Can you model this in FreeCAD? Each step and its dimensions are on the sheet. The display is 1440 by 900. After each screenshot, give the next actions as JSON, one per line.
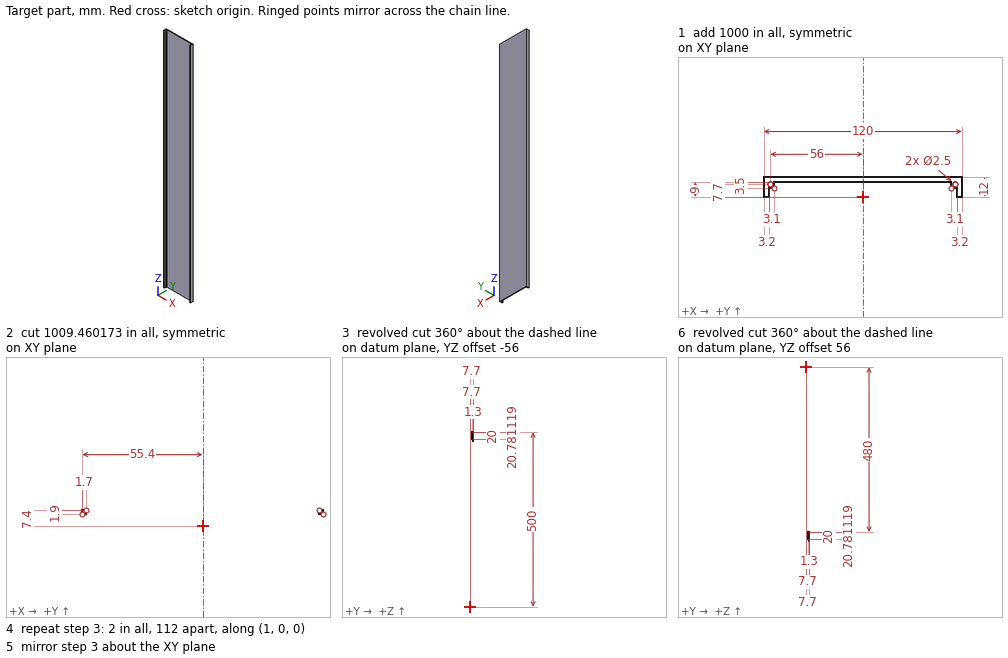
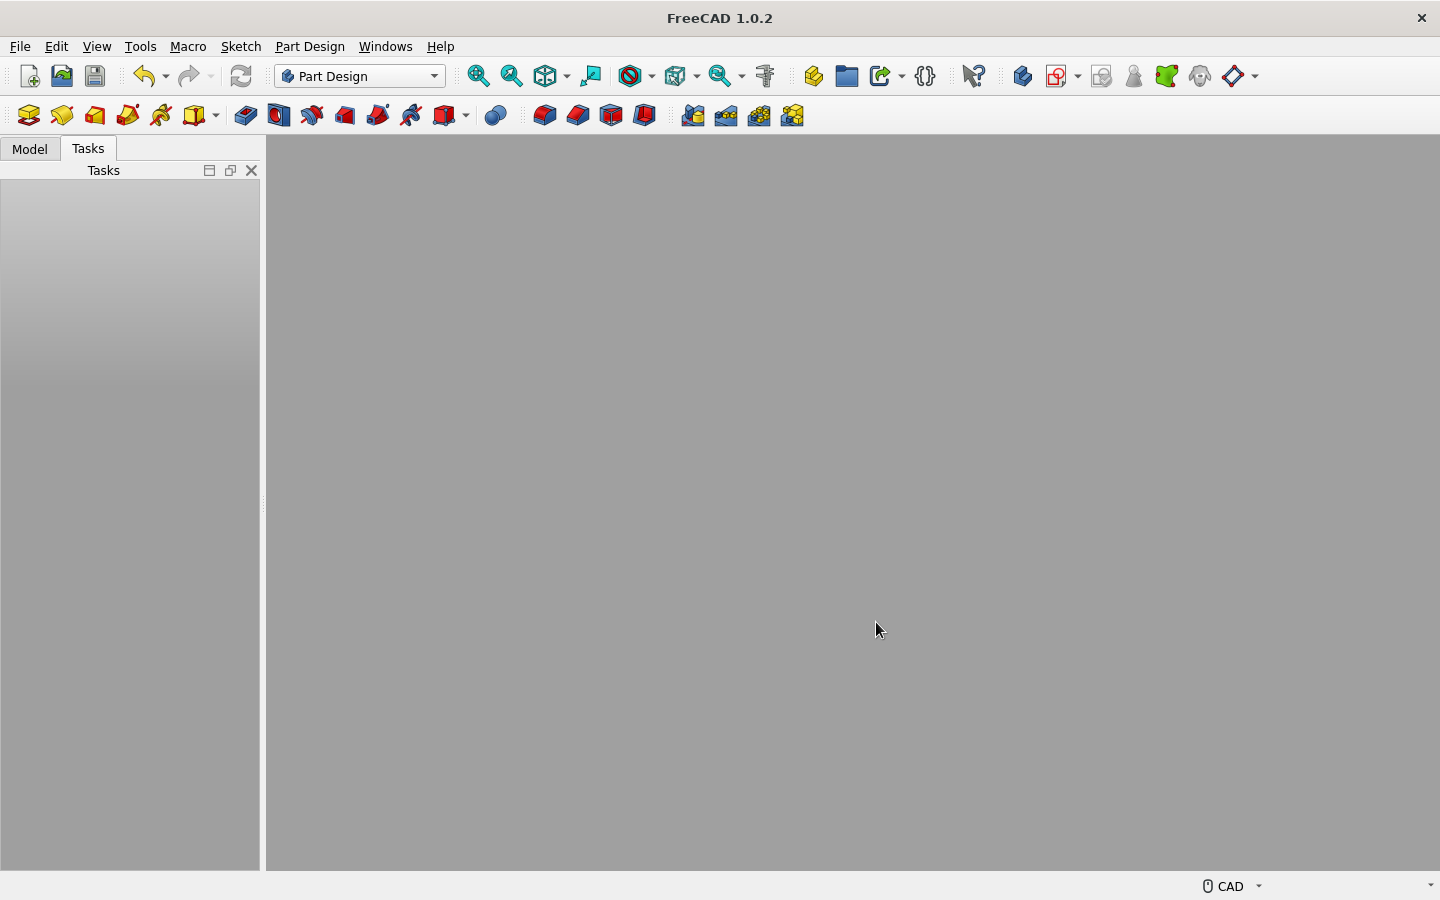
{"action": "left_click", "coordinate": [29, 76]}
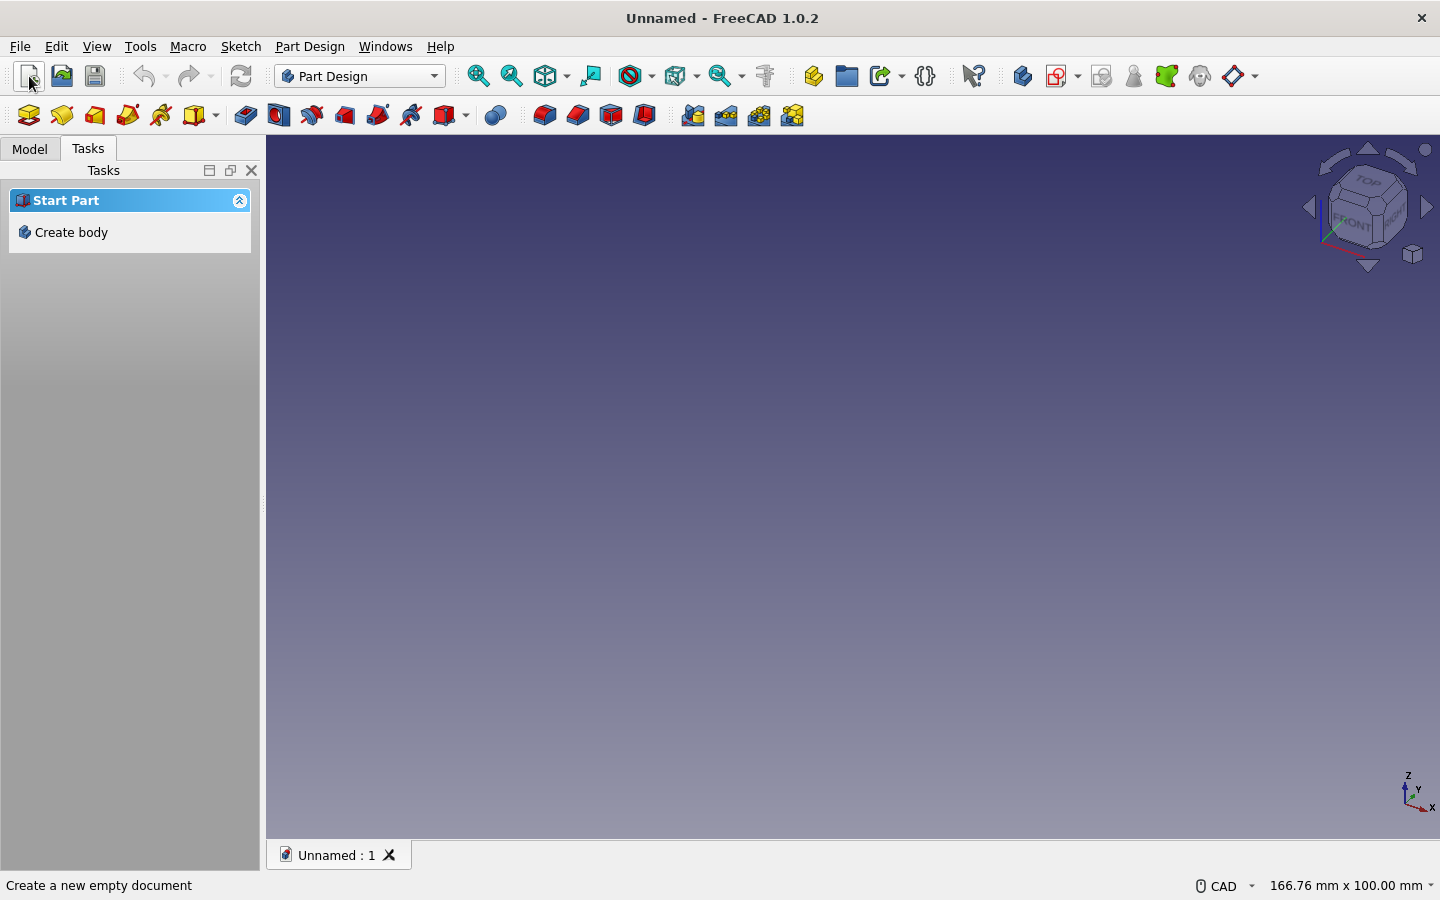
{"action": "left_click", "coordinate": [1056, 76]}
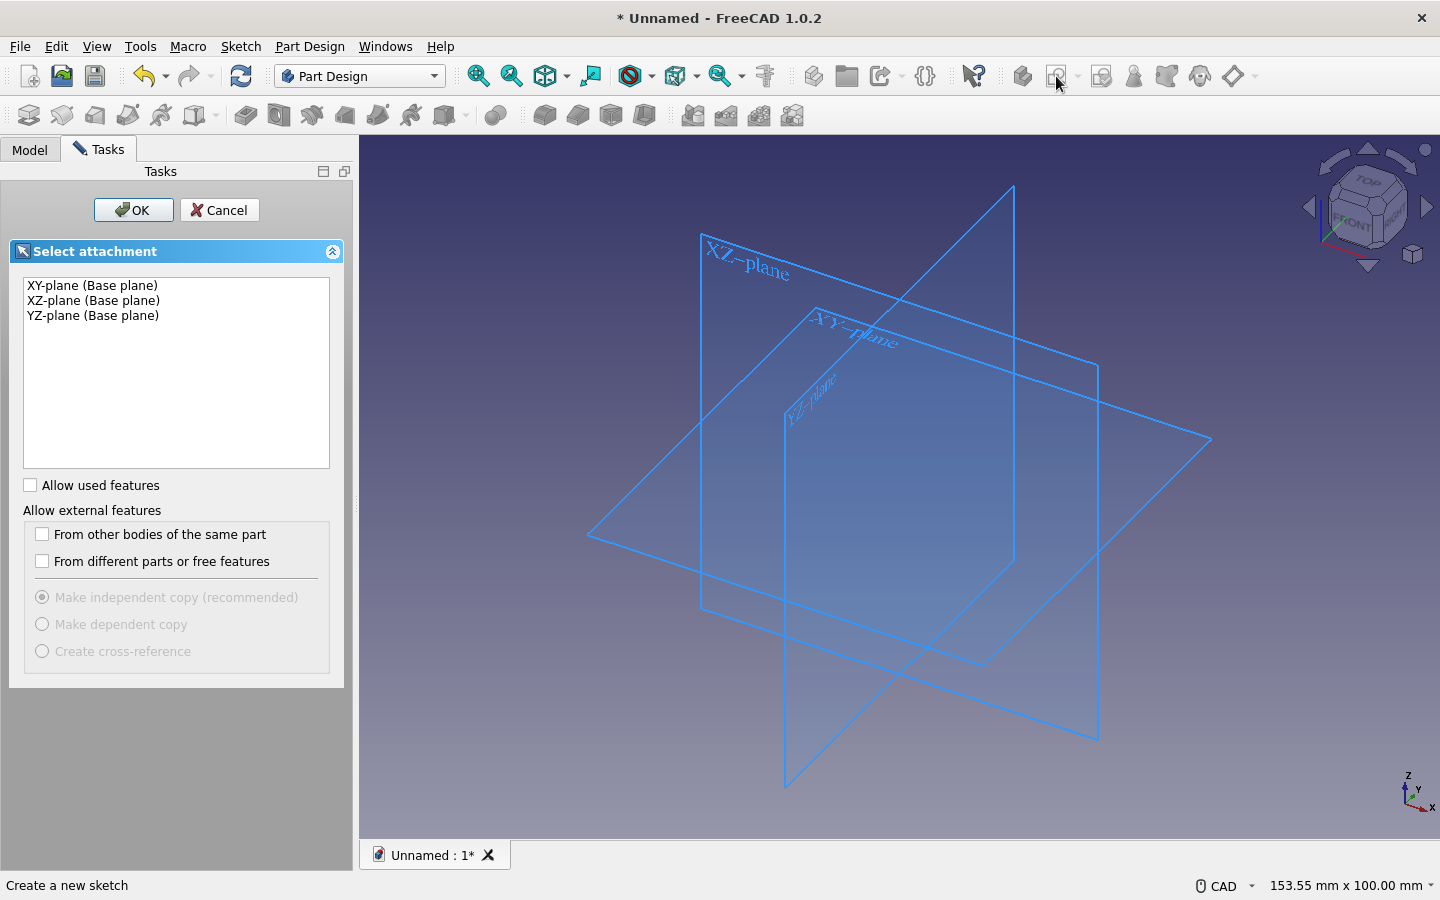
{"action": "left_click", "coordinate": [84, 286]}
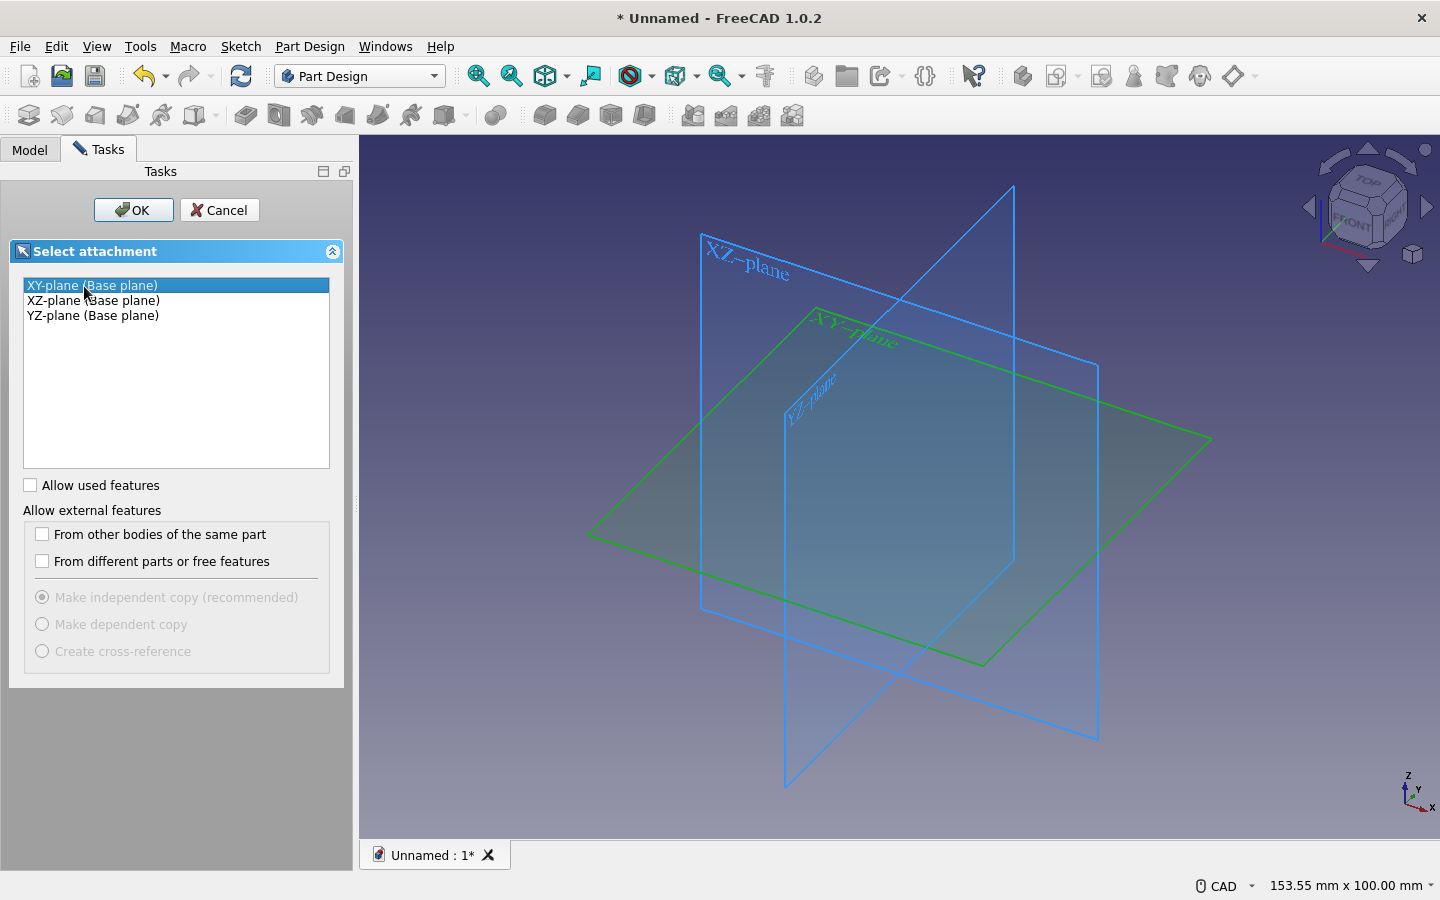
{"action": "left_click", "coordinate": [134, 210]}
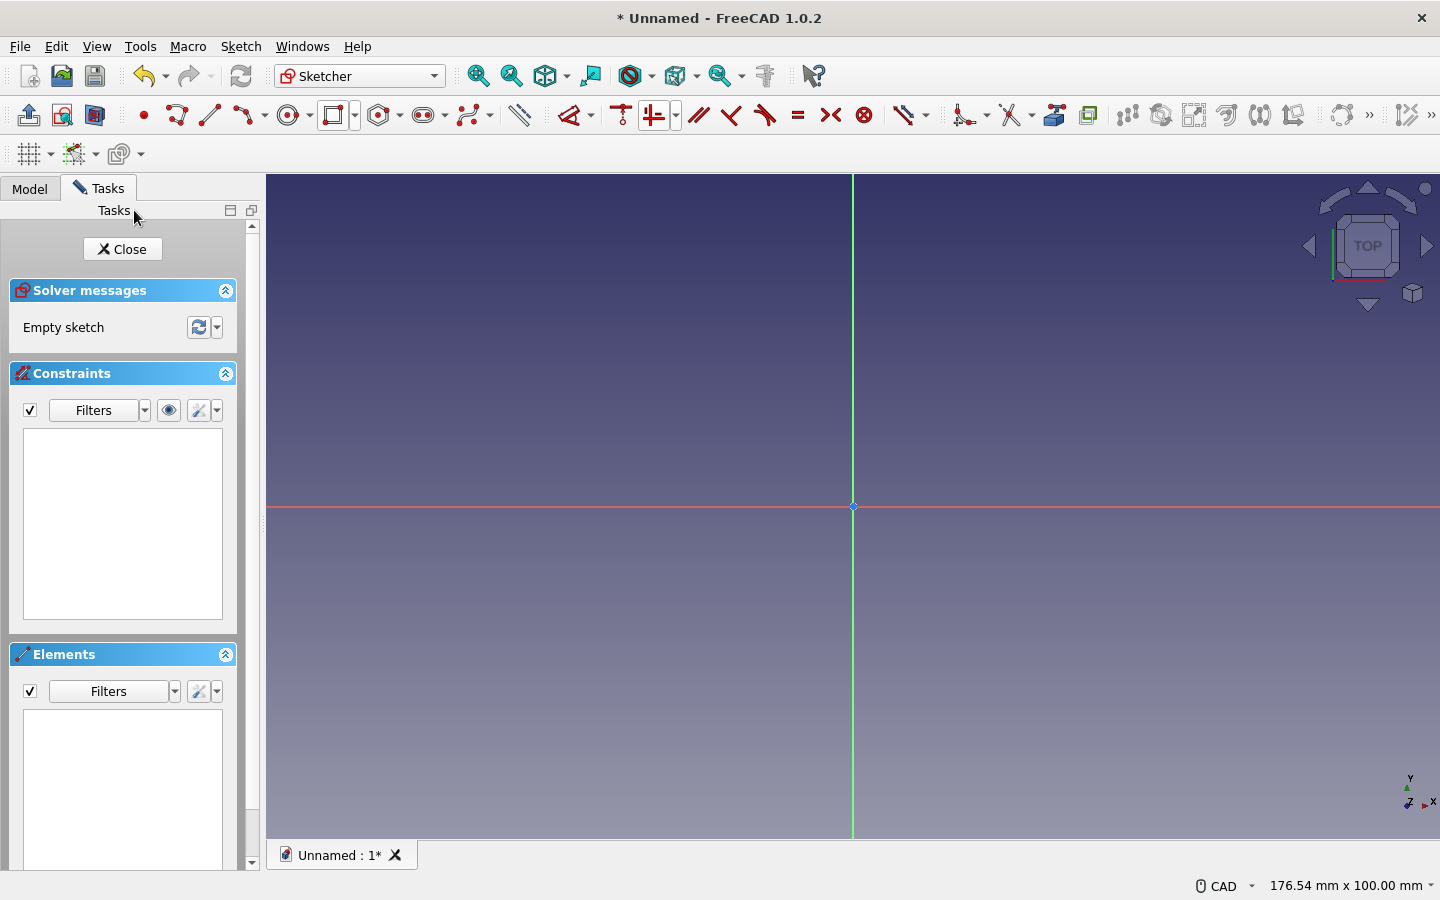
{"action": "scroll", "coordinate": [475, 687], "scroll_direction": "down", "scroll_amount": 1}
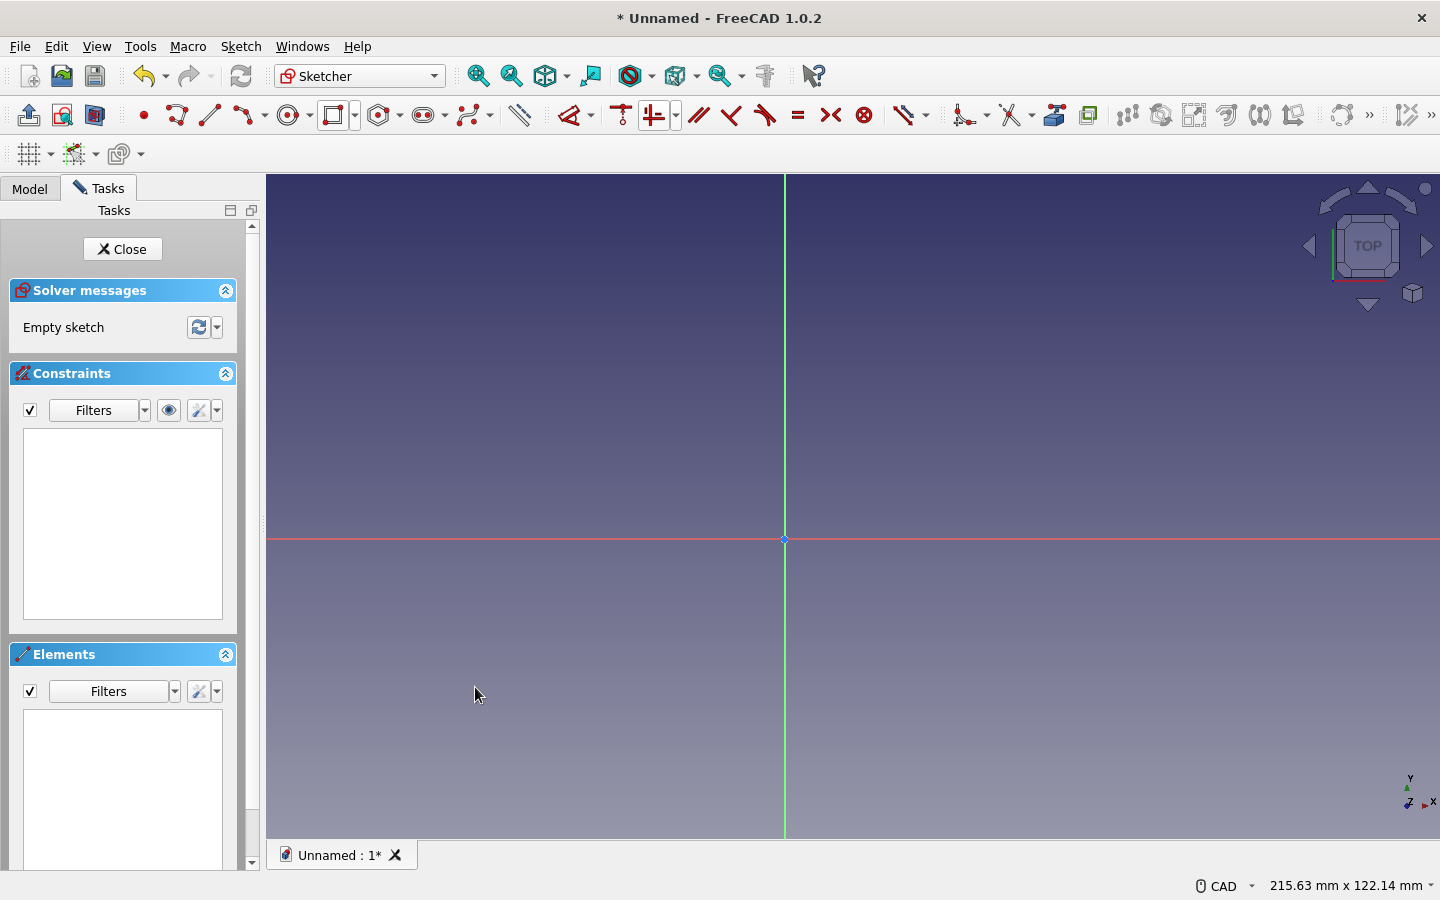
{"action": "key", "text": "g m"}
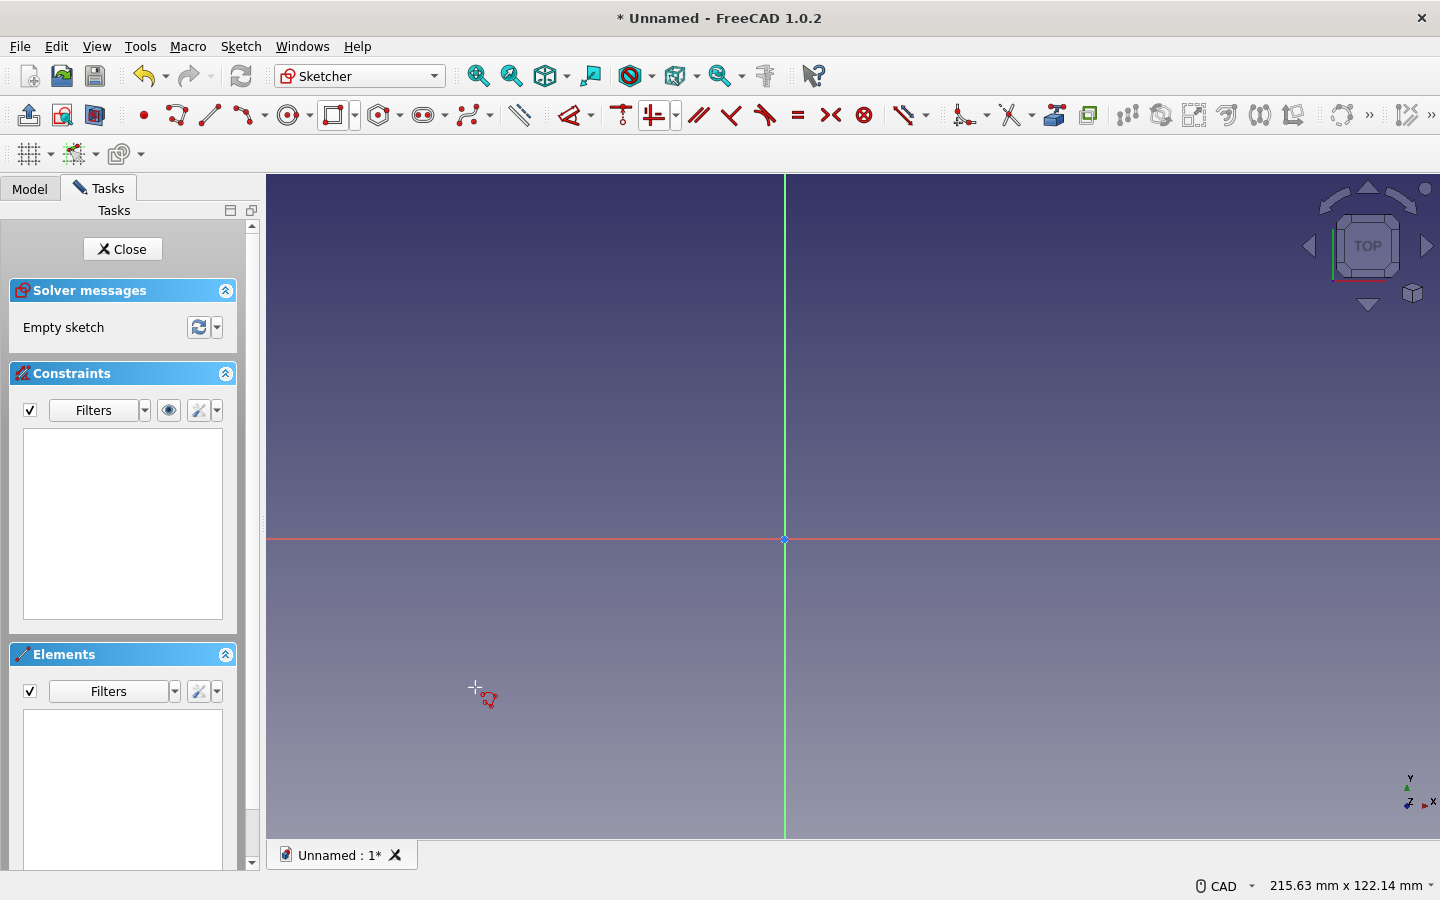
{"action": "left_click", "coordinate": [492, 509]}
{"action": "left_click", "coordinate": [492, 490]}
{"action": "left_click", "coordinate": [1077, 490]}
{"action": "left_click", "coordinate": [1077, 509]}
{"action": "left_click", "coordinate": [1094, 509]}
{"action": "left_click", "coordinate": [1094, 539]}
{"action": "left_click", "coordinate": [1111, 530]}
{"action": "left_click", "coordinate": [1111, 474]}
{"action": "left_click", "coordinate": [458, 474]}
{"action": "left_click", "coordinate": [458, 539]}
{"action": "left_click", "coordinate": [475, 530]}
{"action": "left_click", "coordinate": [475, 509]}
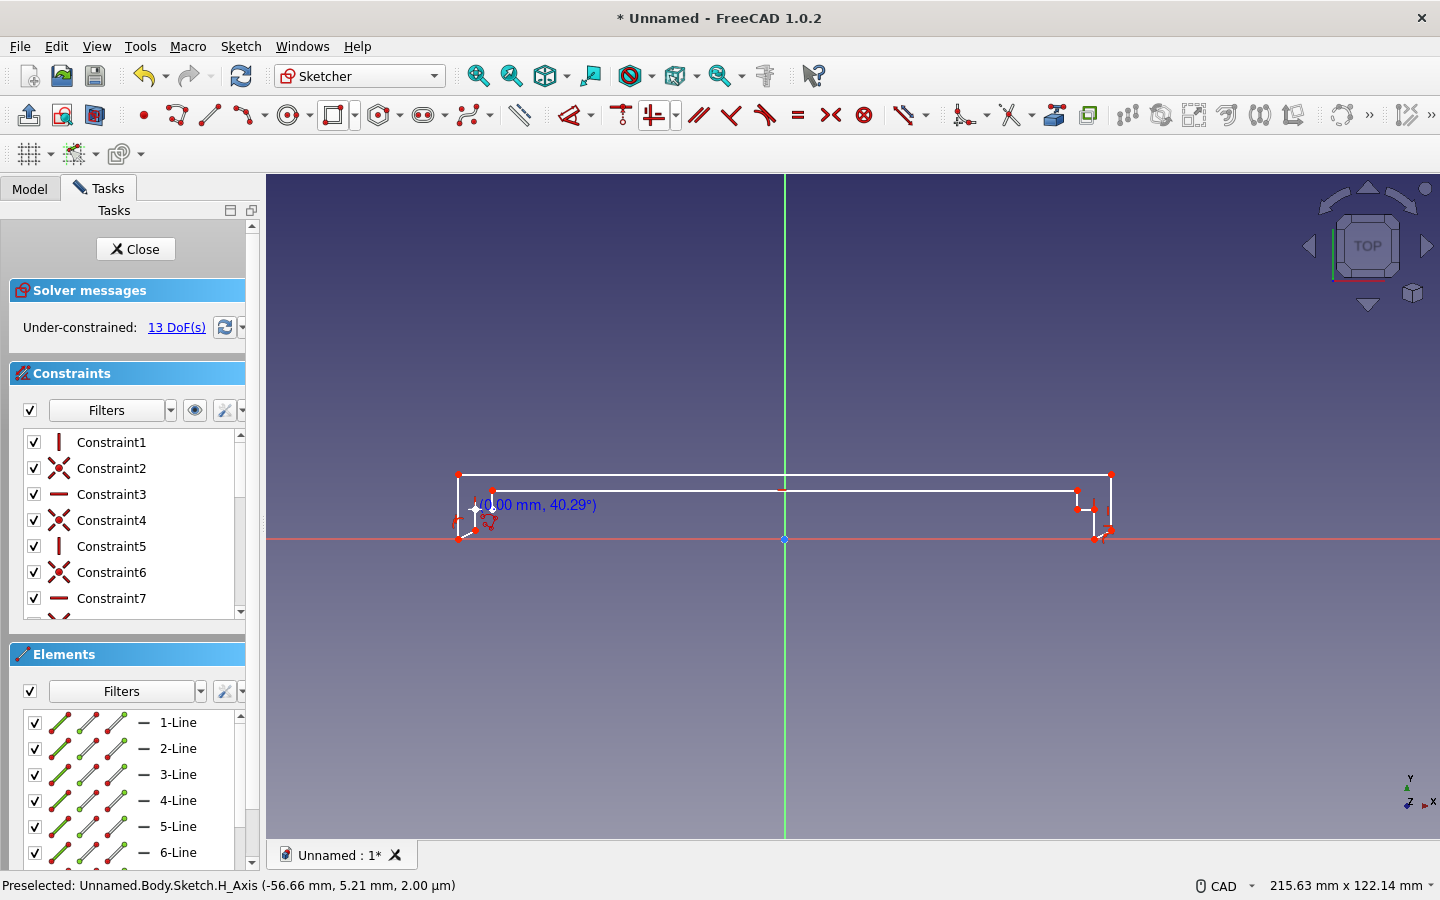
{"action": "scroll", "coordinate": [492, 509], "scroll_direction": "up", "scroll_amount": 3}